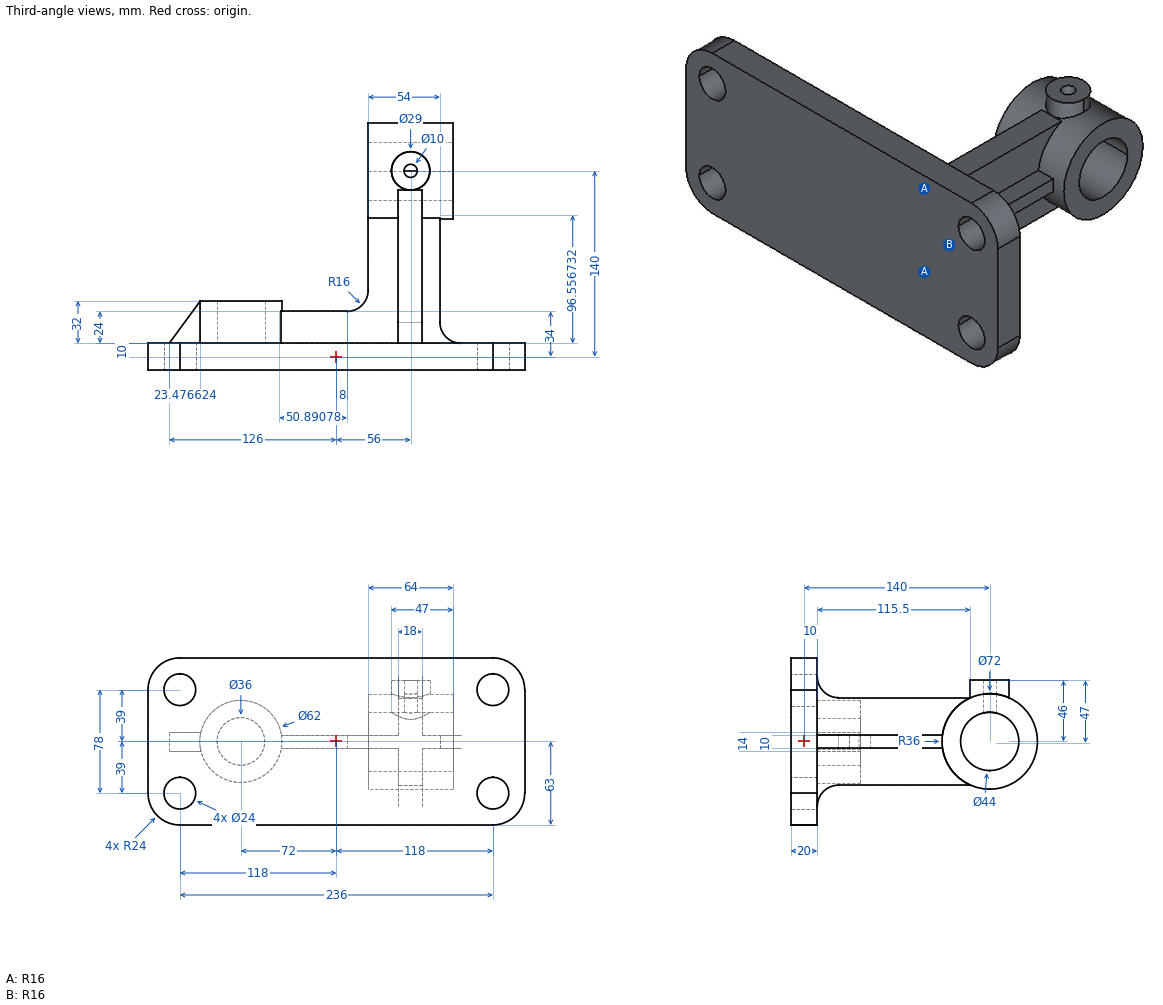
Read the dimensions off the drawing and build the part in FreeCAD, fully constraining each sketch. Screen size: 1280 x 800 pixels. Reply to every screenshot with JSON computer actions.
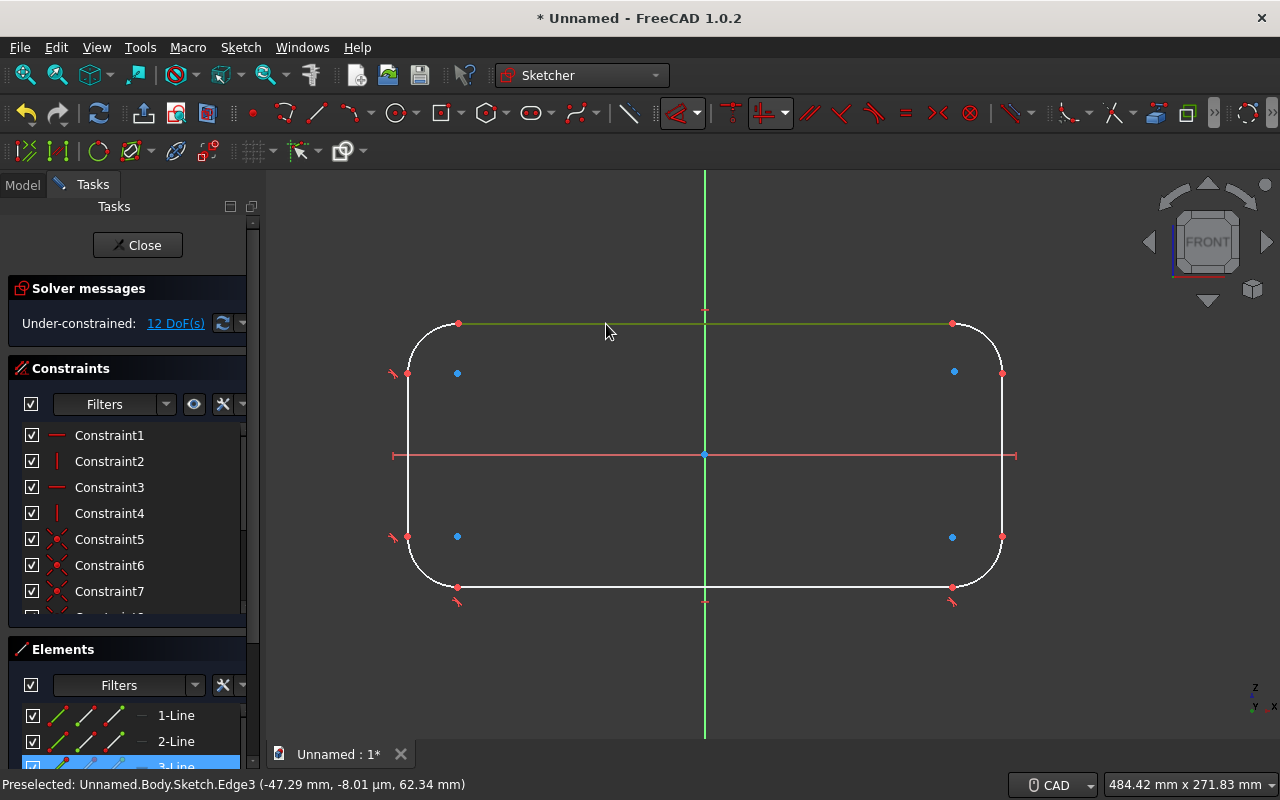
{"action": "left_click", "coordinate": [435, 329]}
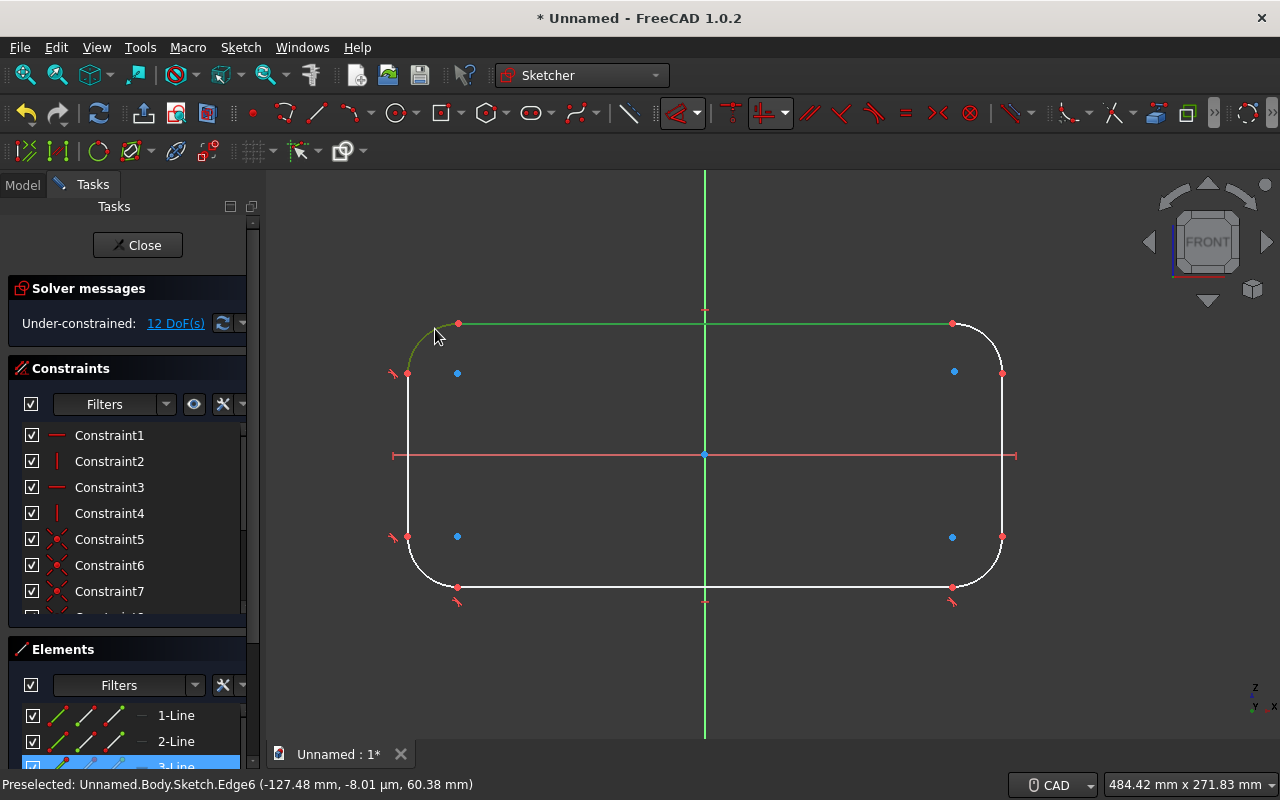
{"action": "left_click", "coordinate": [874, 114]}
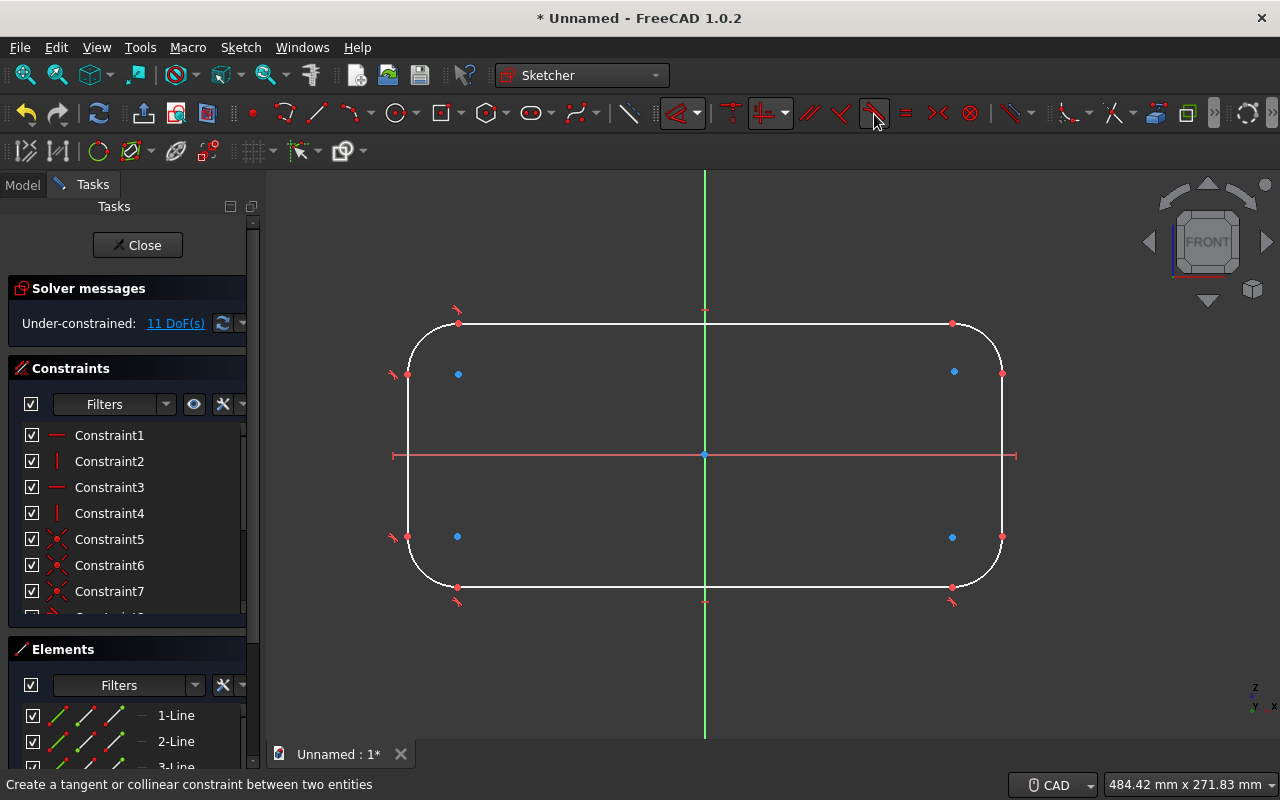
{"action": "left_click", "coordinate": [606, 324]}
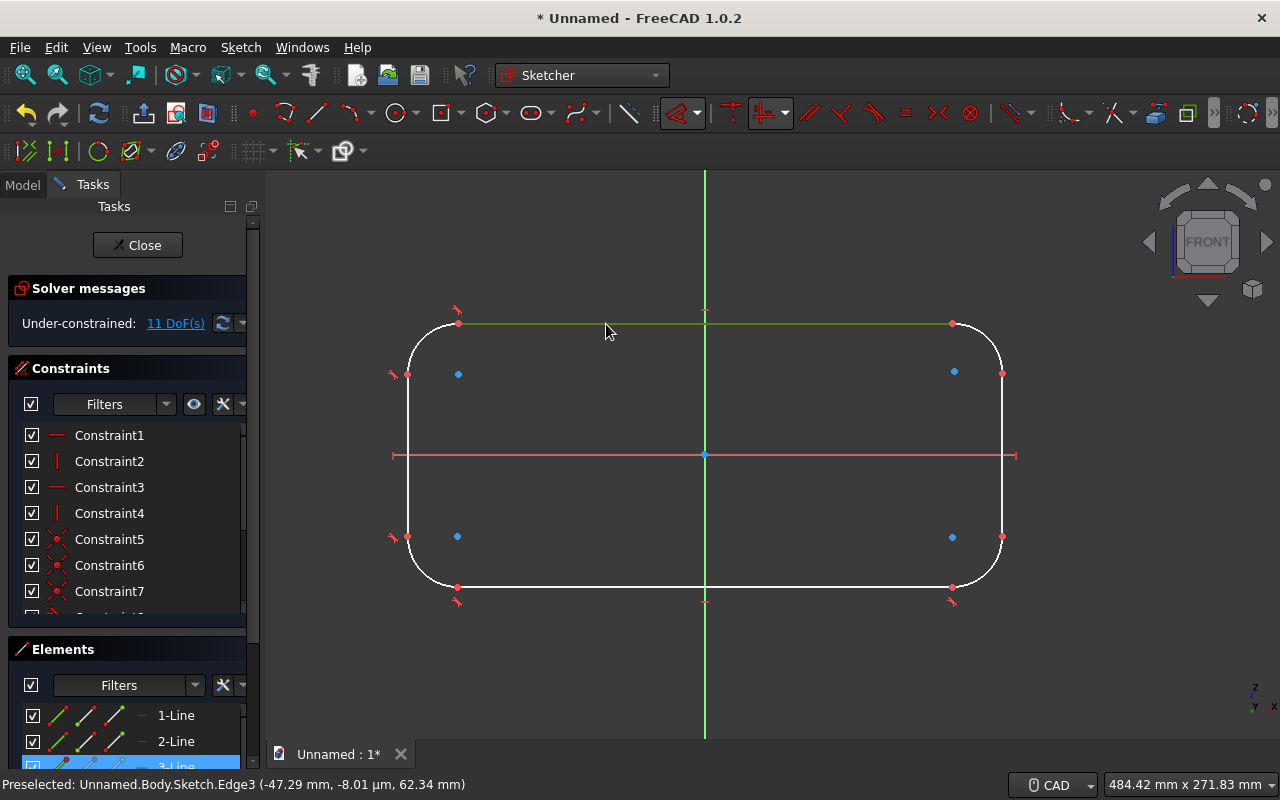
{"action": "left_click", "coordinate": [997, 351]}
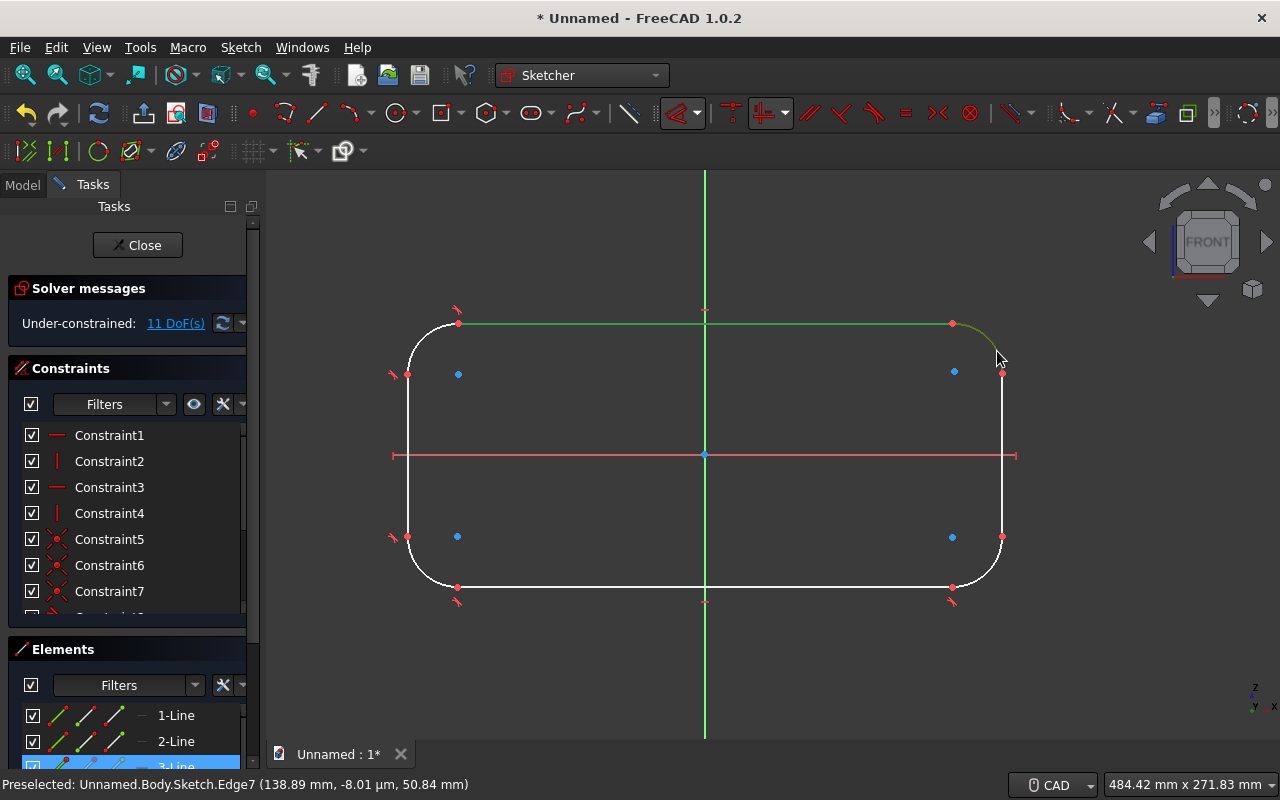
{"action": "left_click", "coordinate": [874, 114]}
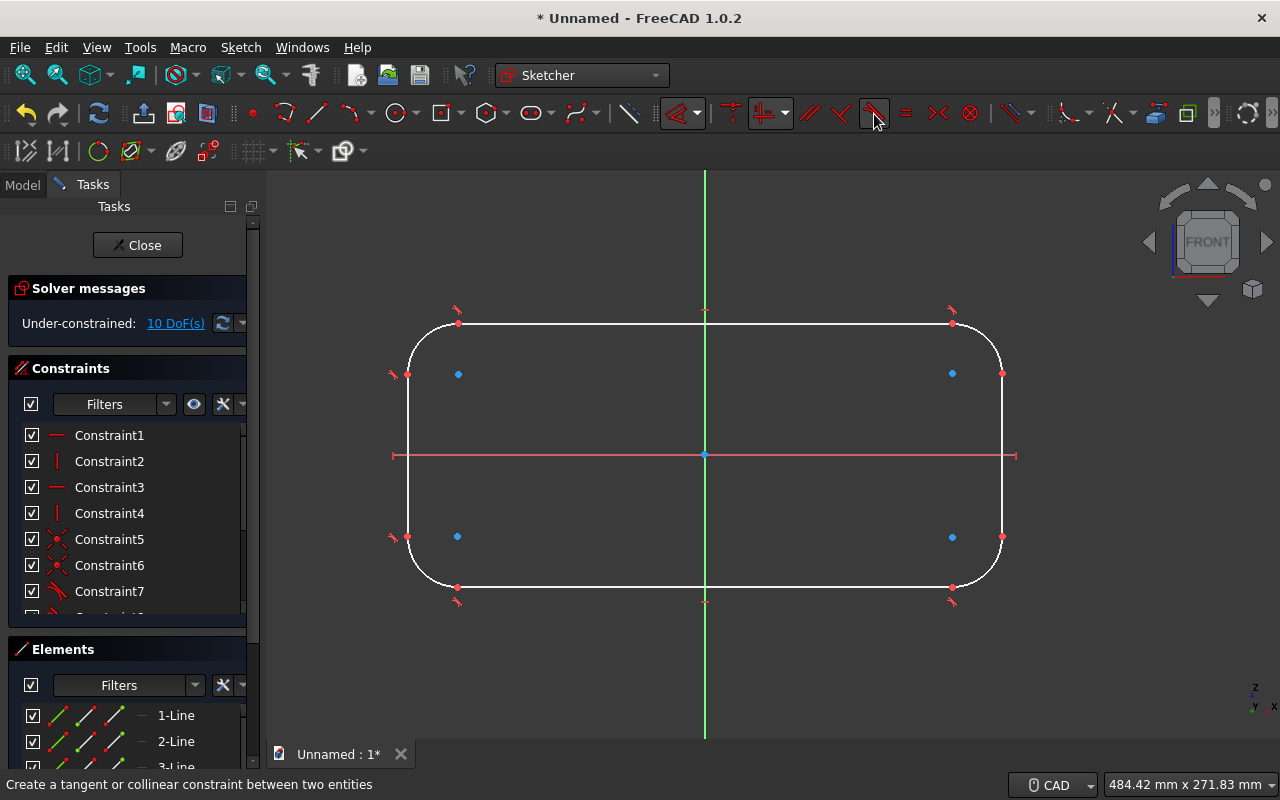
{"action": "left_click", "coordinate": [1002, 423]}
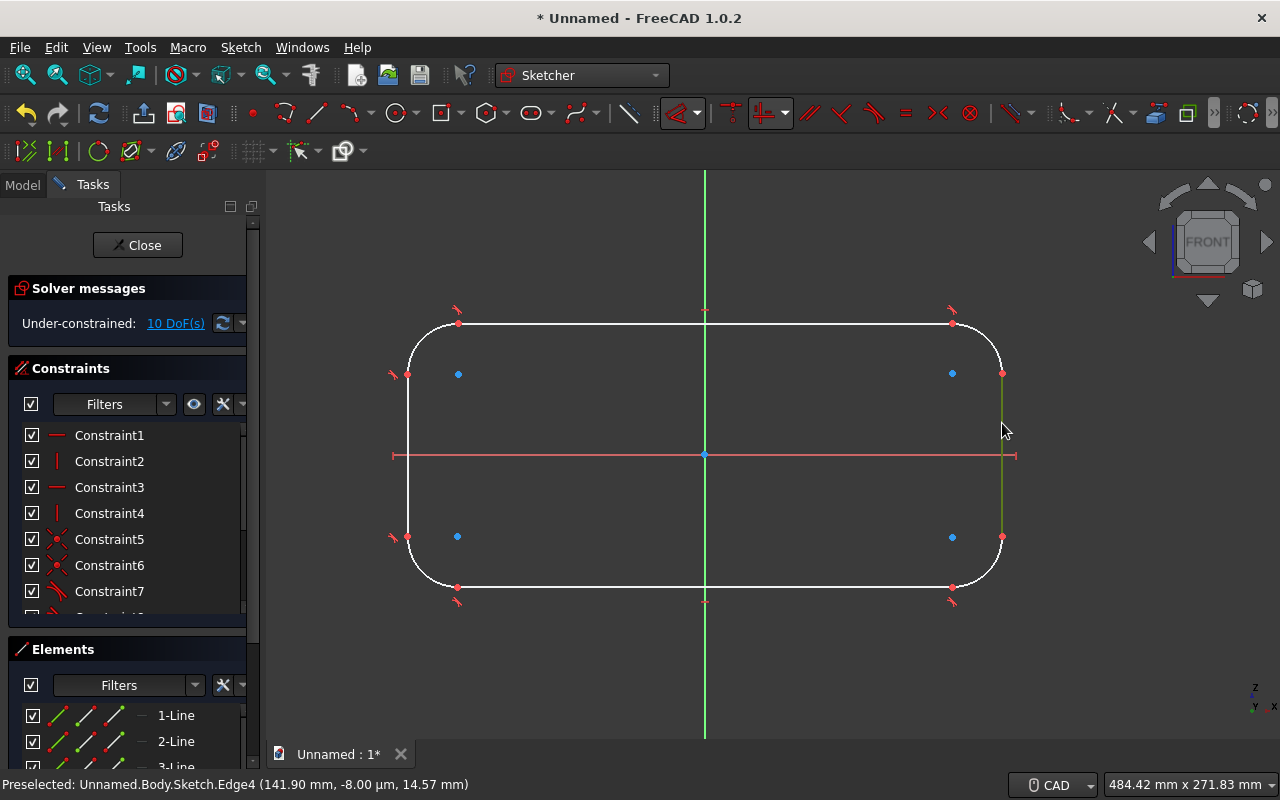
{"action": "left_click", "coordinate": [997, 351]}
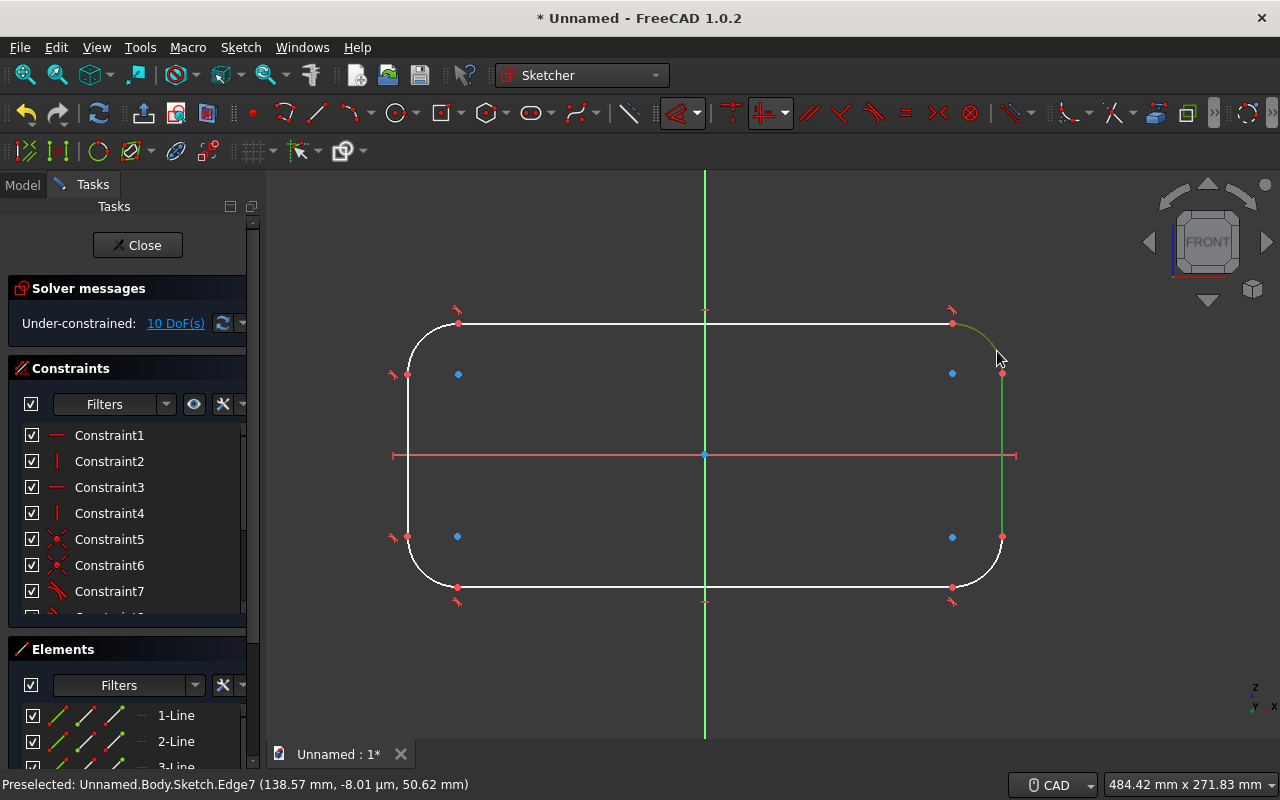
{"action": "left_click", "coordinate": [874, 114]}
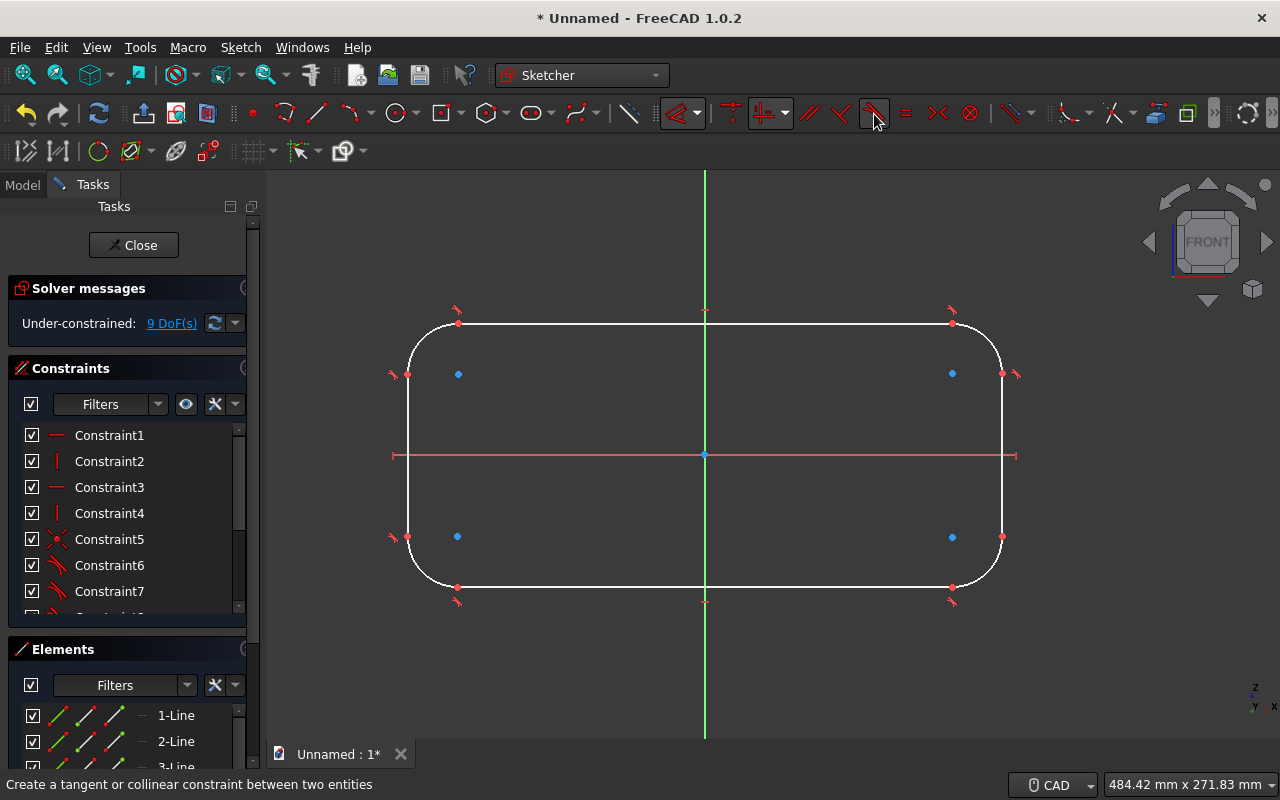
{"action": "left_click", "coordinate": [1002, 423]}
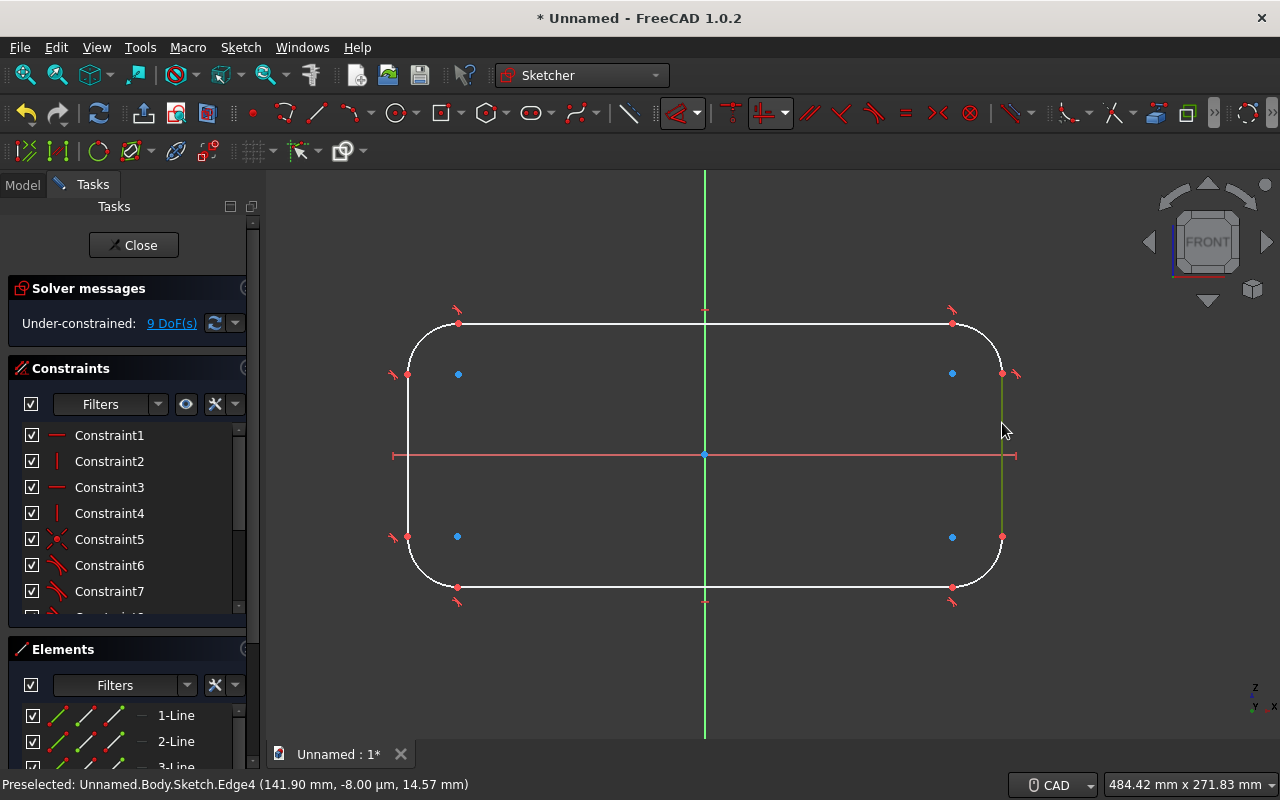
{"action": "left_click", "coordinate": [975, 582]}